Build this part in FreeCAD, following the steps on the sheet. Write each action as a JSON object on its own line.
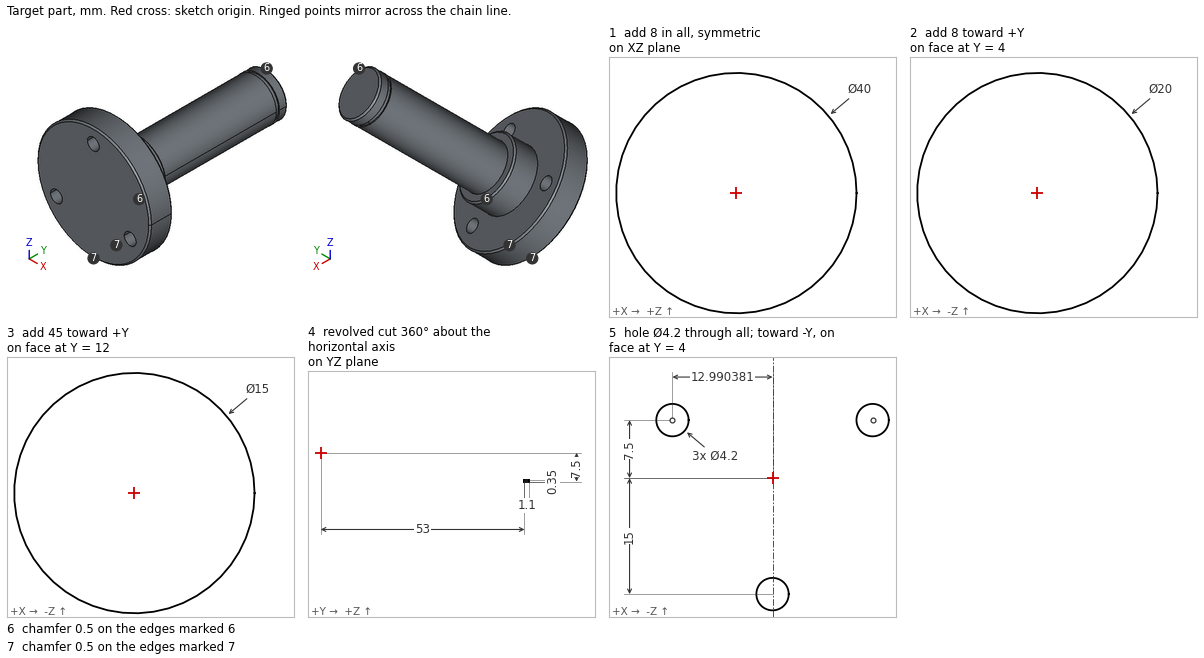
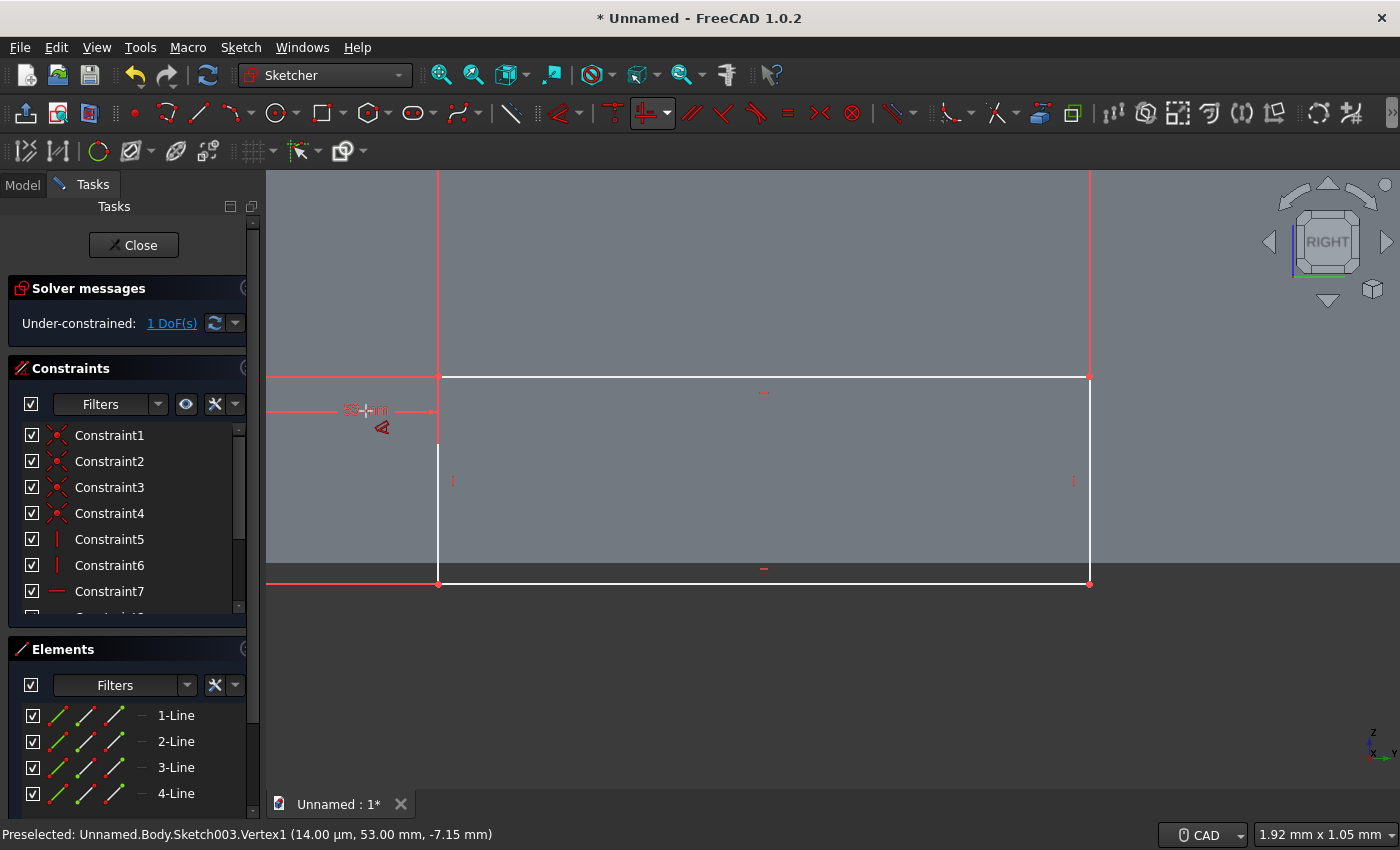
{"action": "left_click", "coordinate": [438, 584]}
{"action": "left_click", "coordinate": [472, 391]}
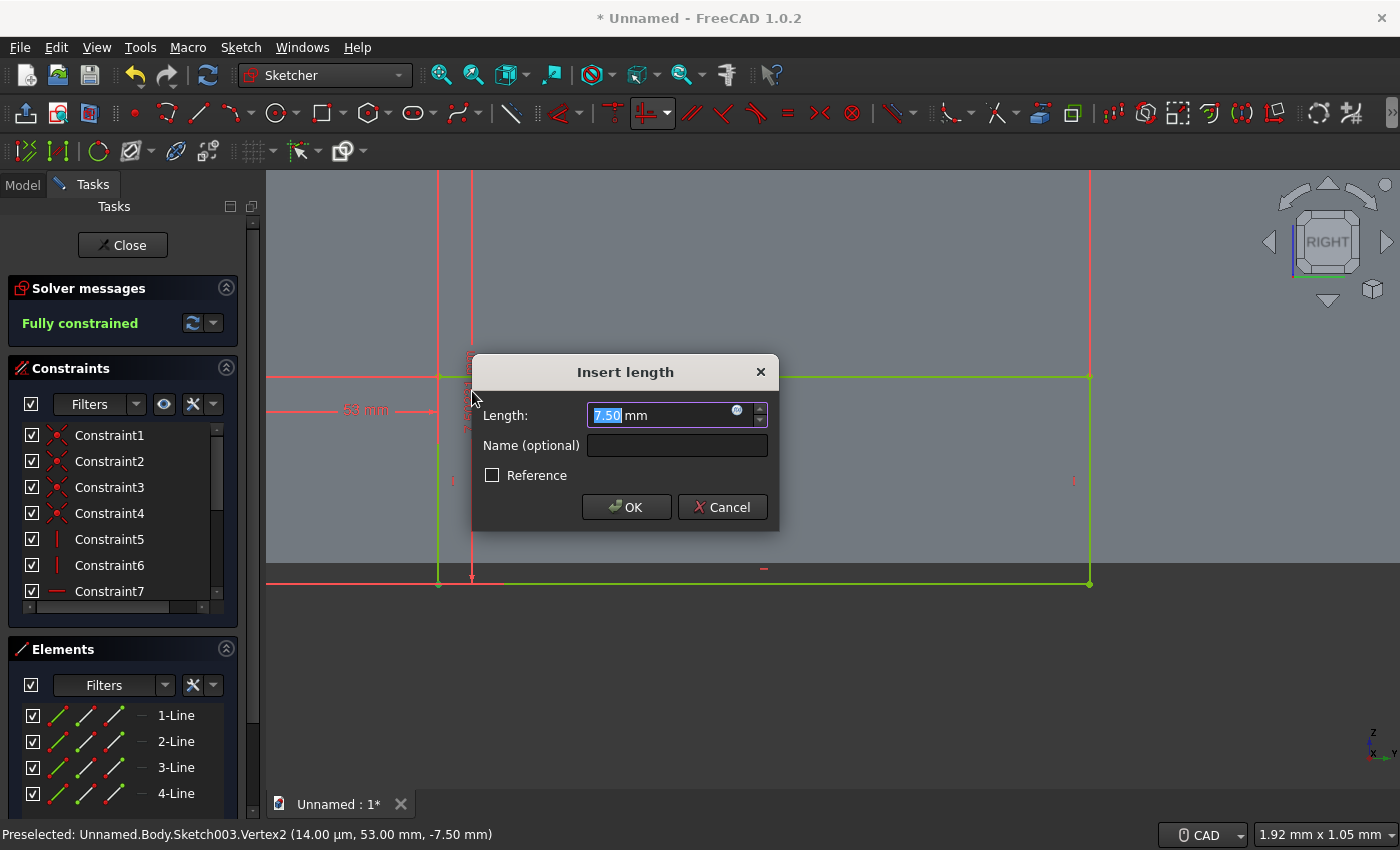
{"action": "type", "text": "7.5"}
{"action": "key", "text": "Return"}
{"action": "key", "text": "Escape"}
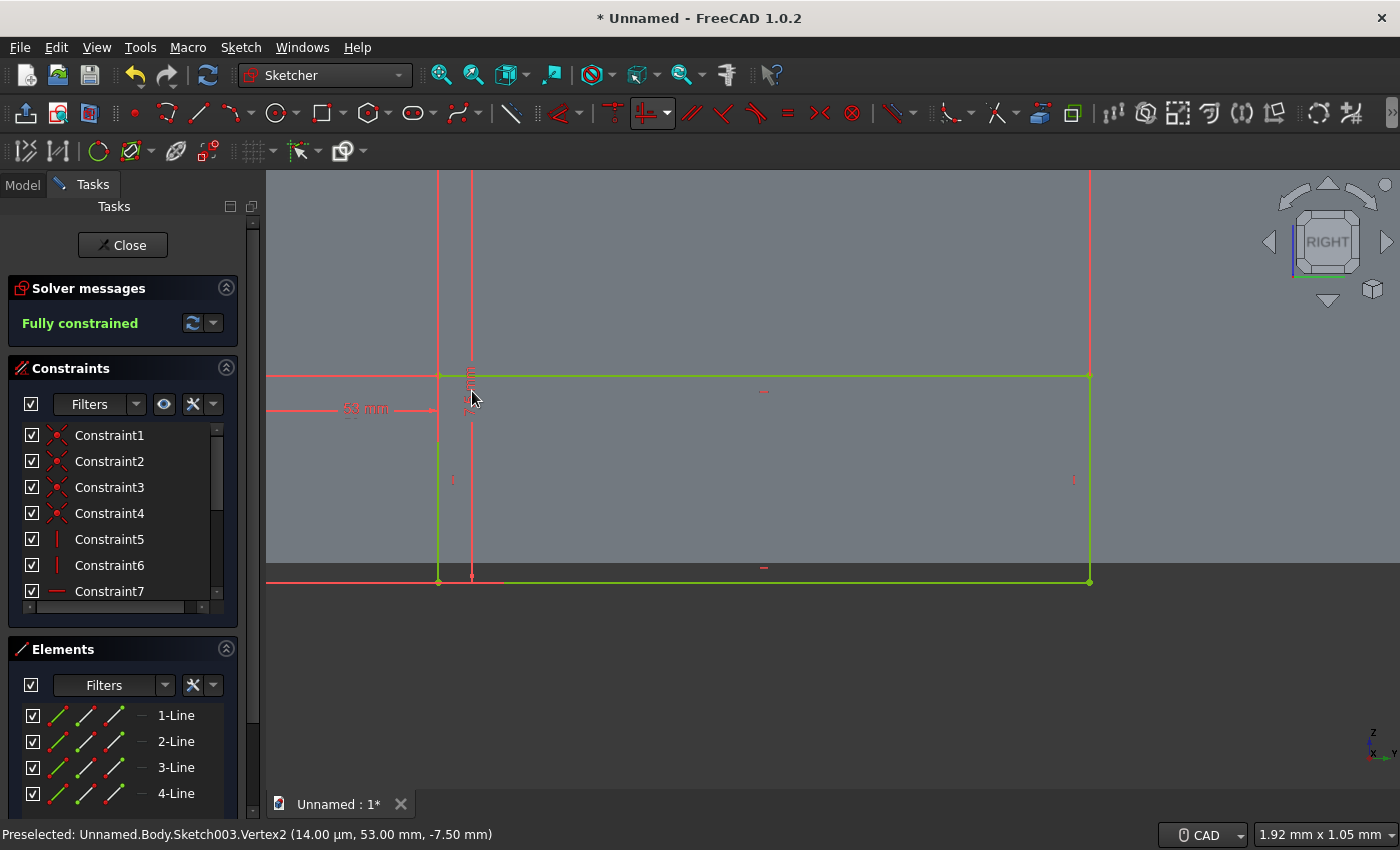
{"action": "left_click", "coordinate": [123, 245]}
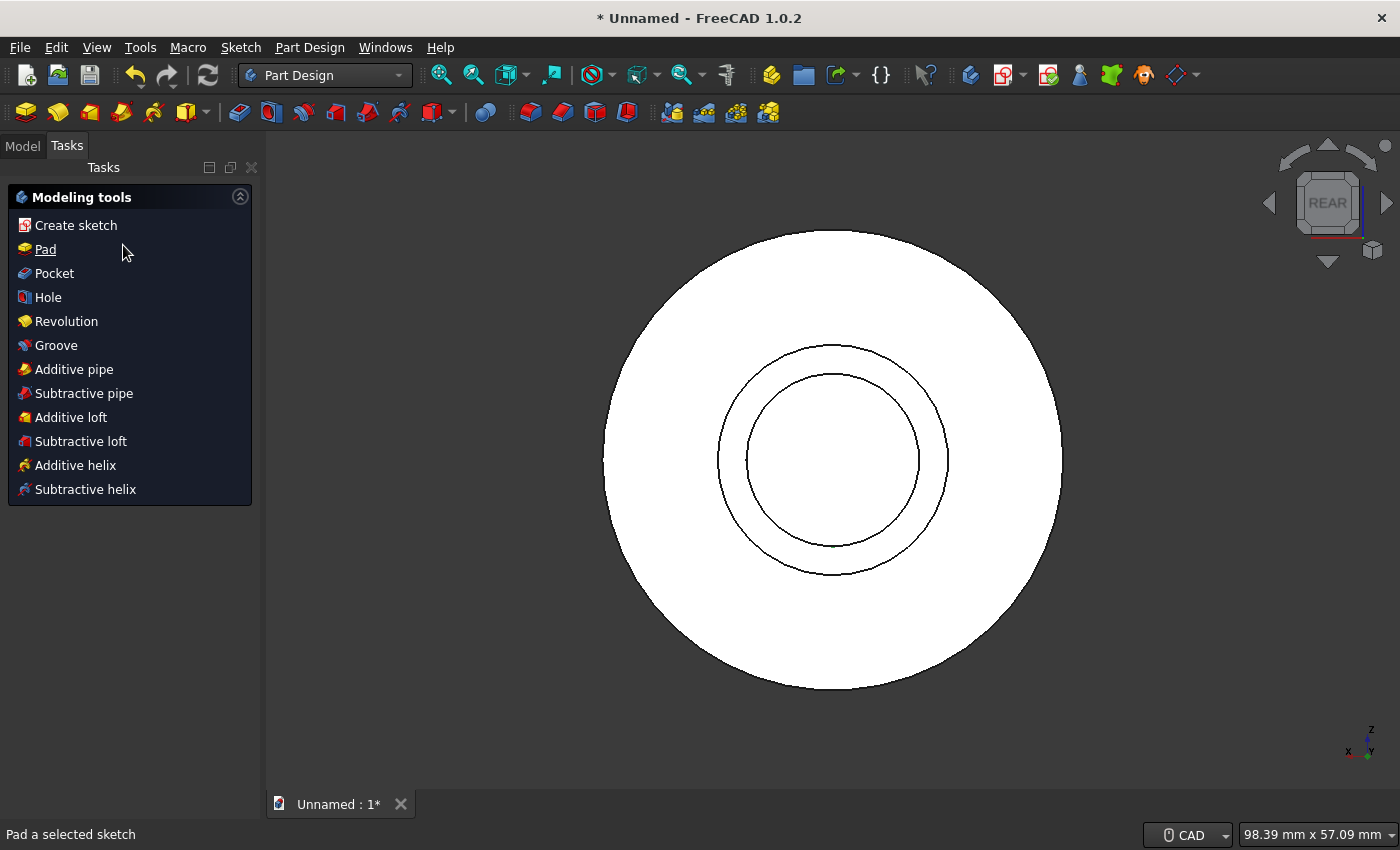
{"action": "left_click", "coordinate": [304, 112]}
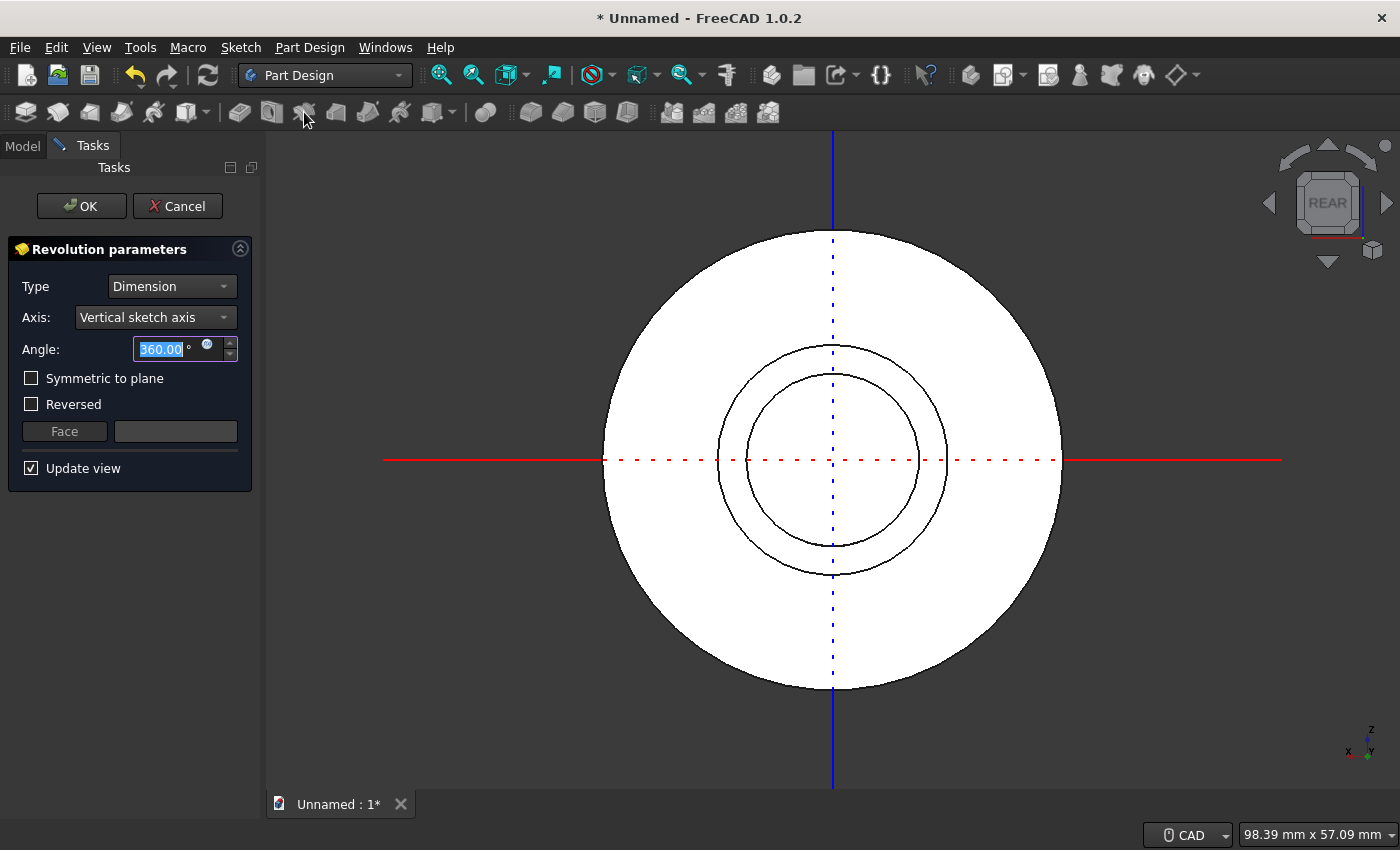
{"action": "left_click", "coordinate": [156, 318]}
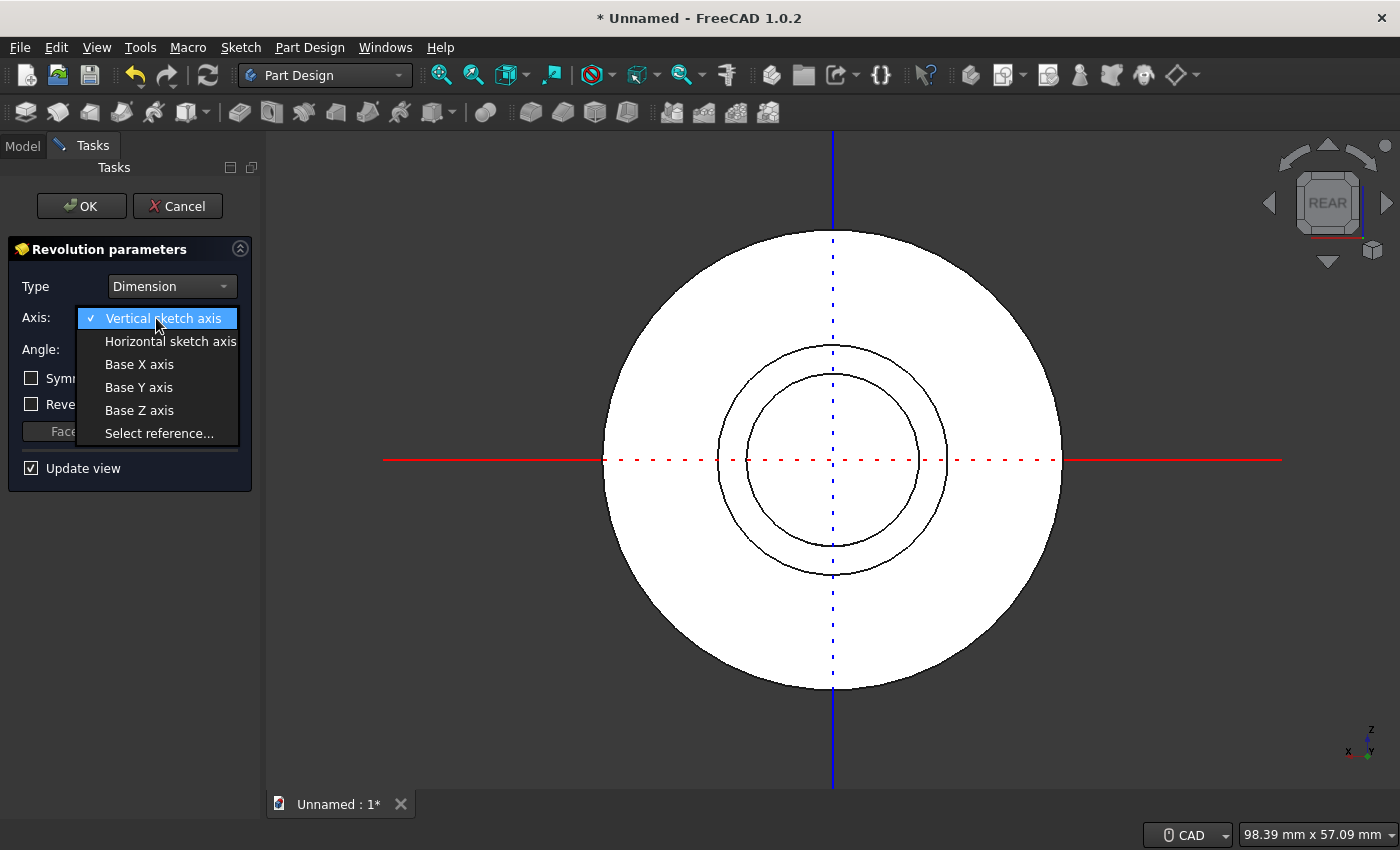
{"action": "left_click", "coordinate": [156, 342]}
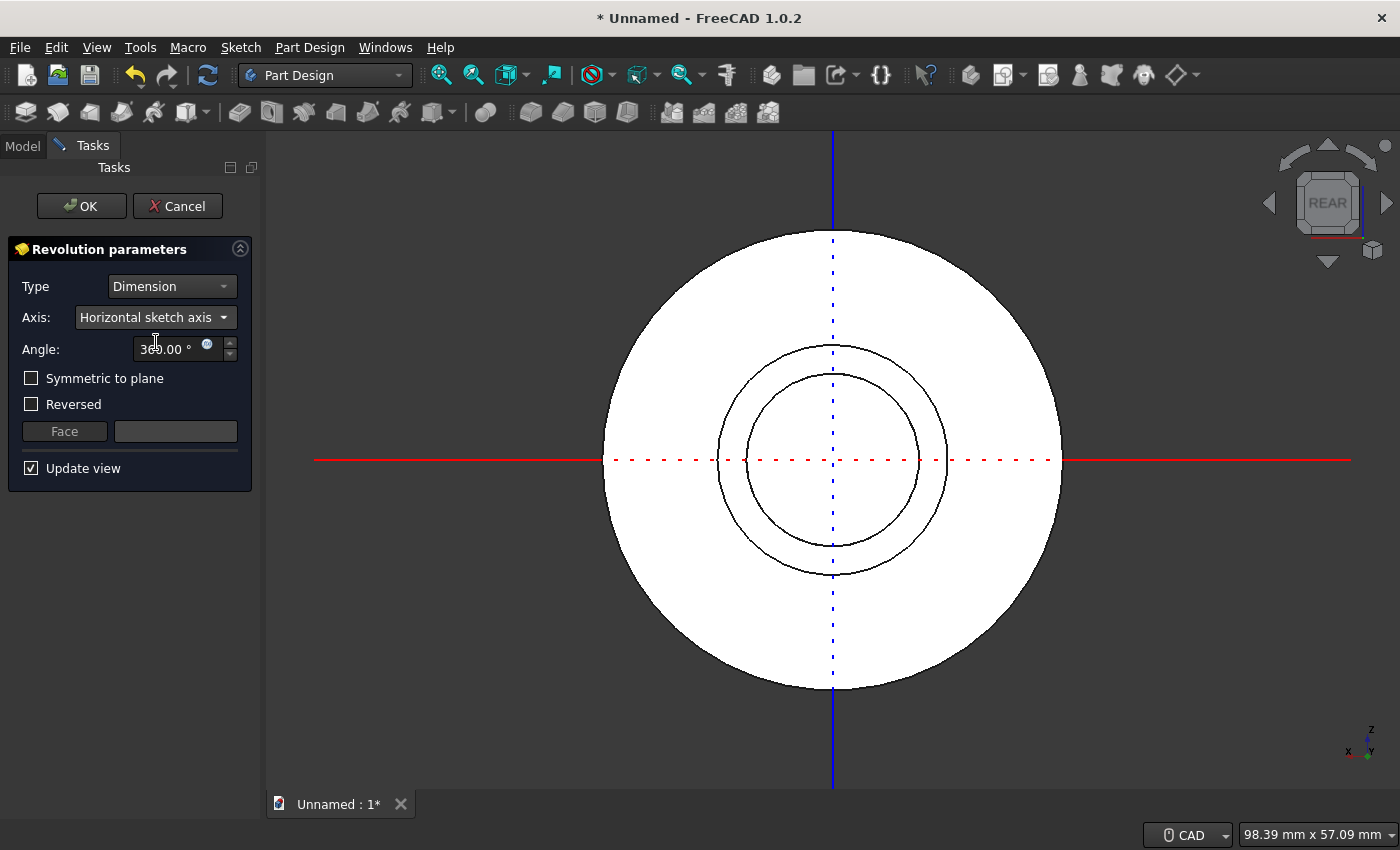
{"action": "left_click", "coordinate": [82, 206]}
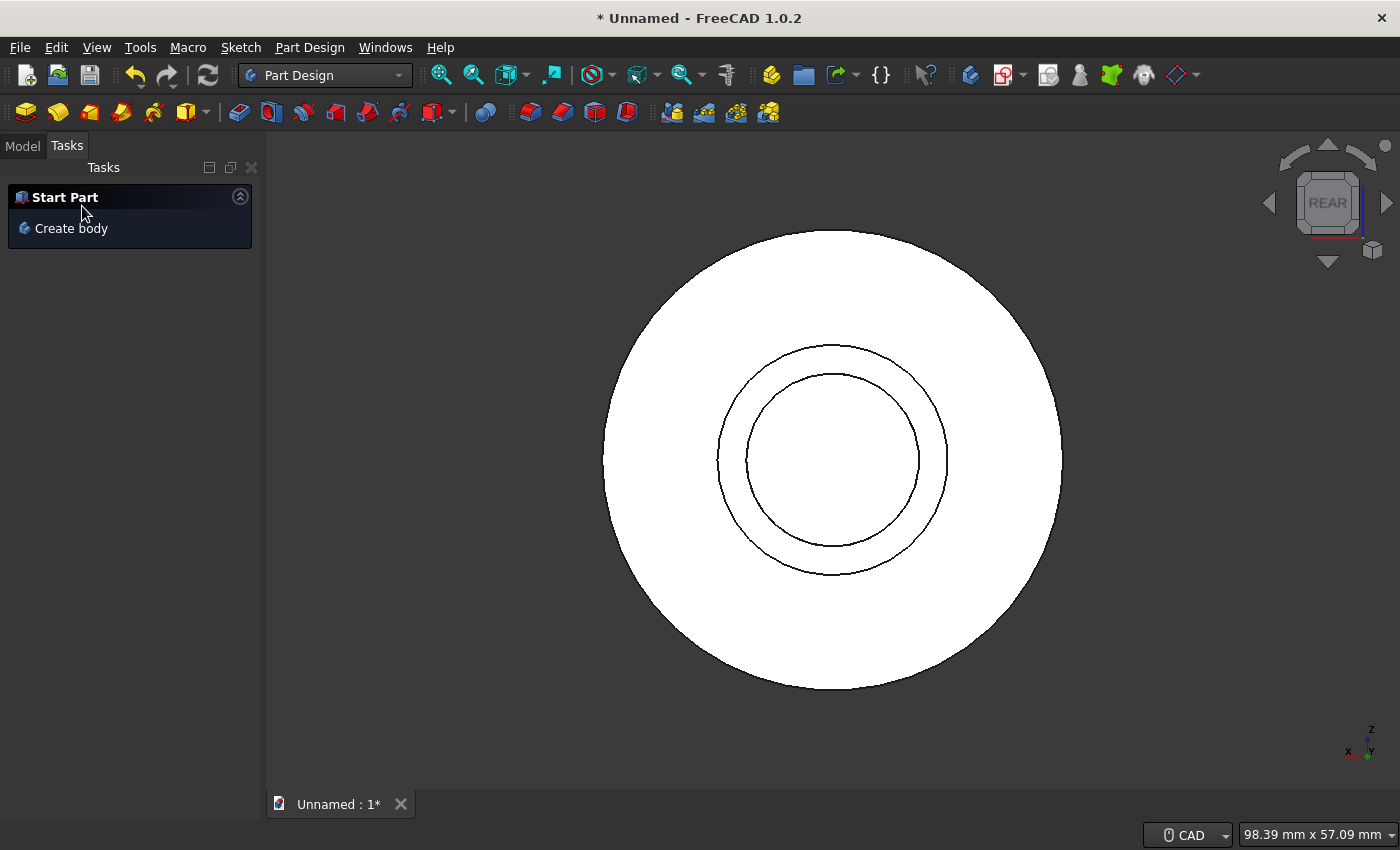
{"action": "left_click", "coordinate": [701, 591]}